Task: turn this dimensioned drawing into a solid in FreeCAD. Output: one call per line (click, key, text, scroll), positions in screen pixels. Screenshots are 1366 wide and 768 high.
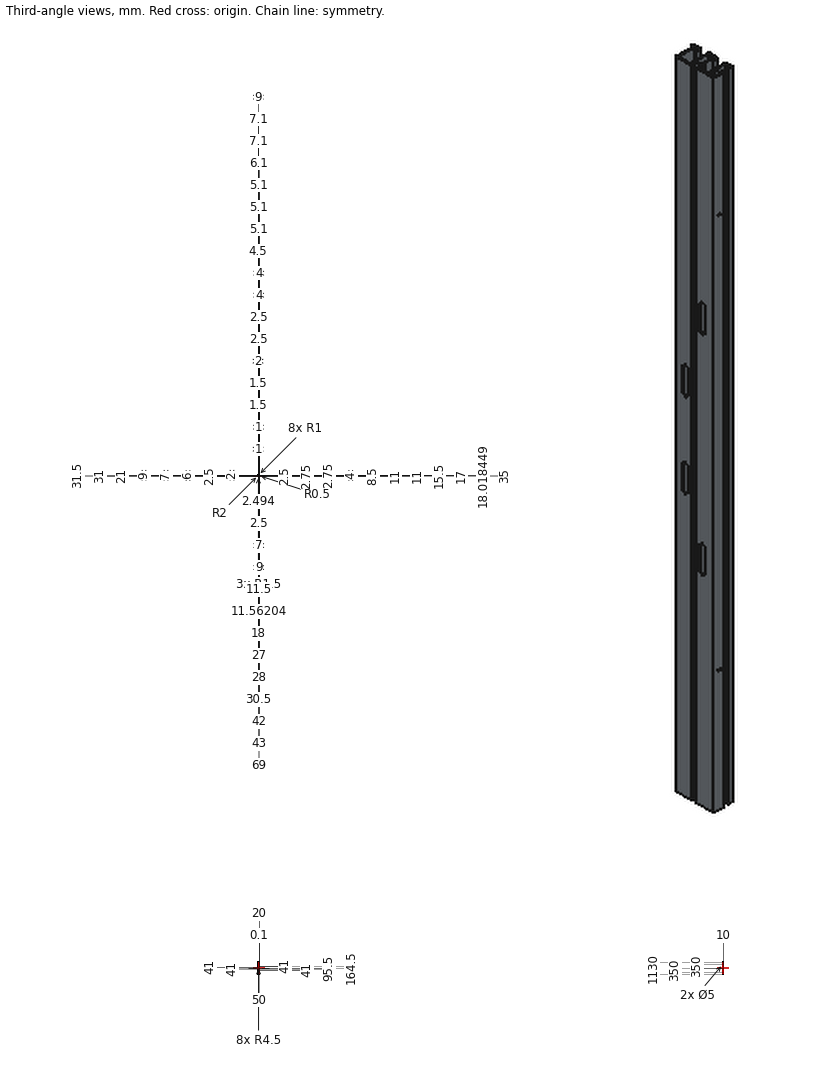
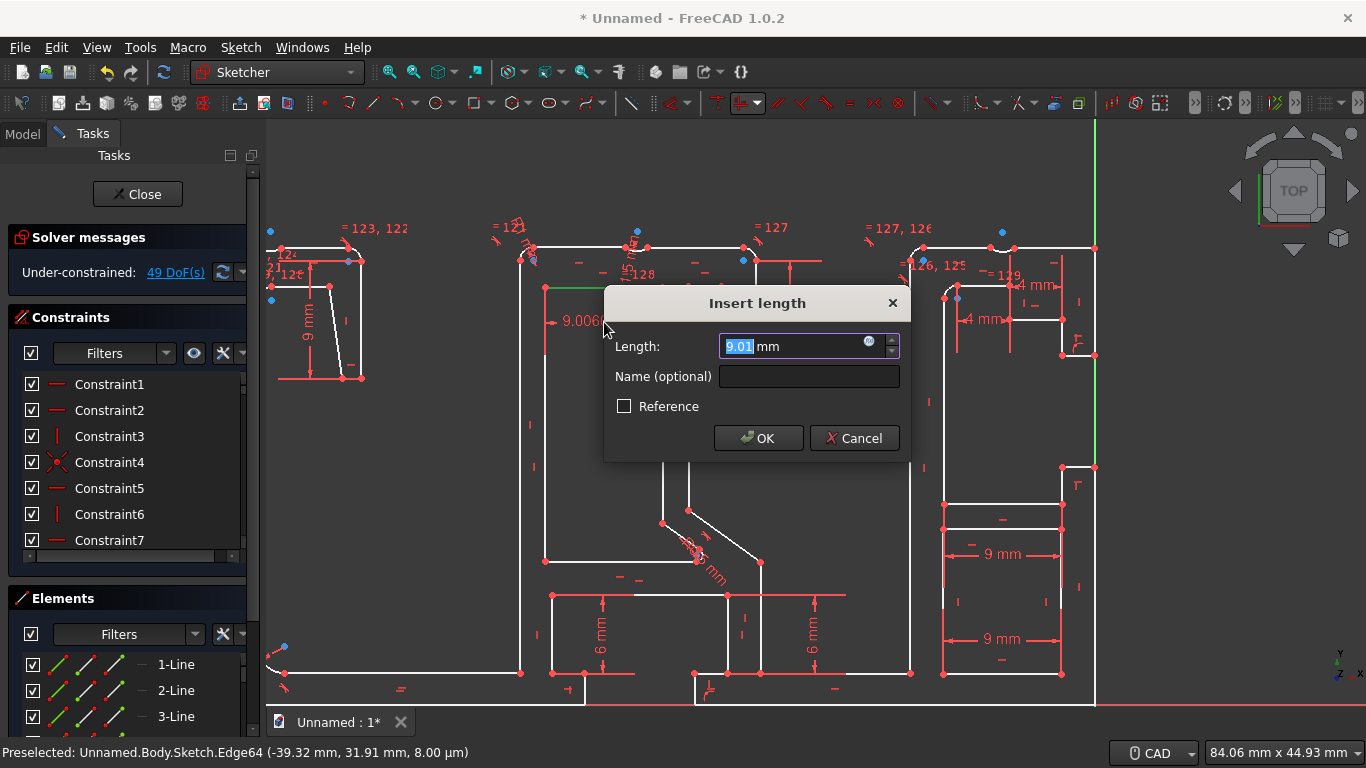
text(9)
key(Return)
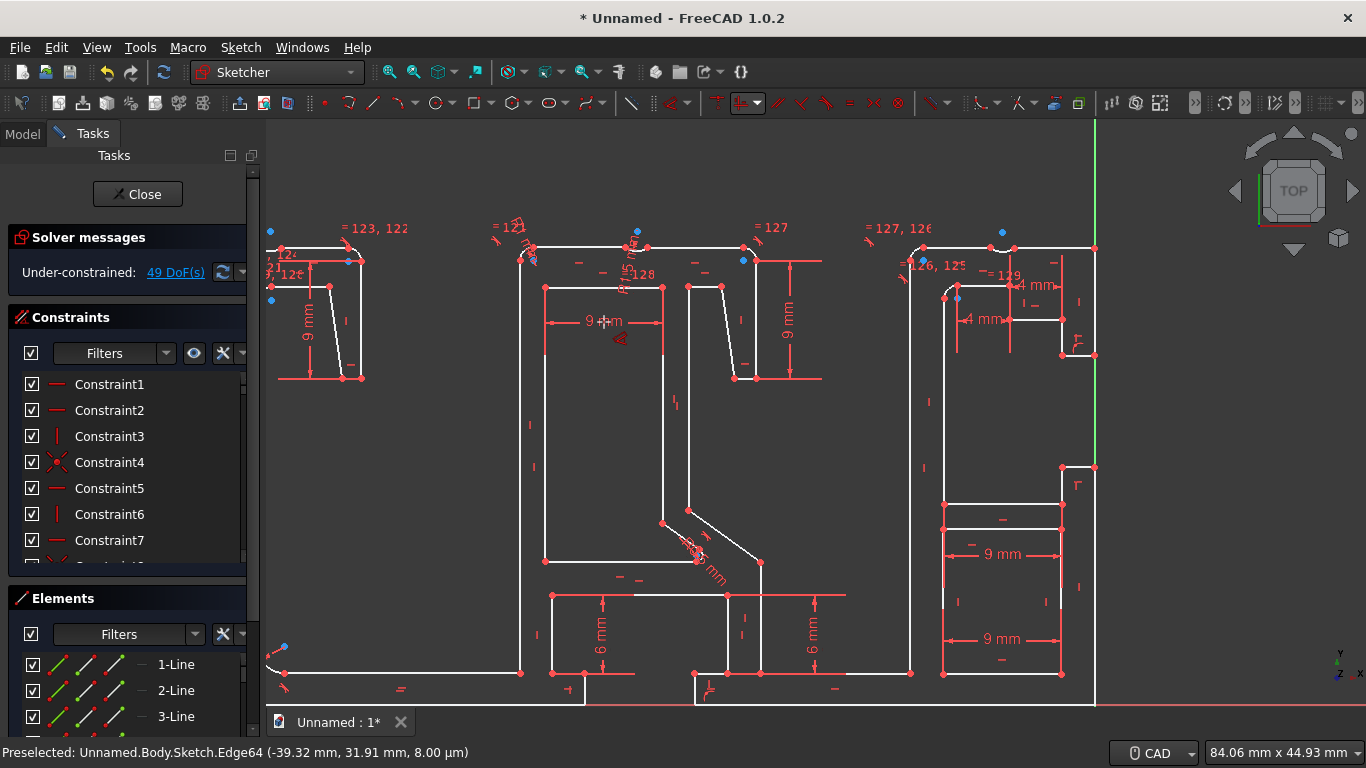
click(449, 673)
click(407, 639)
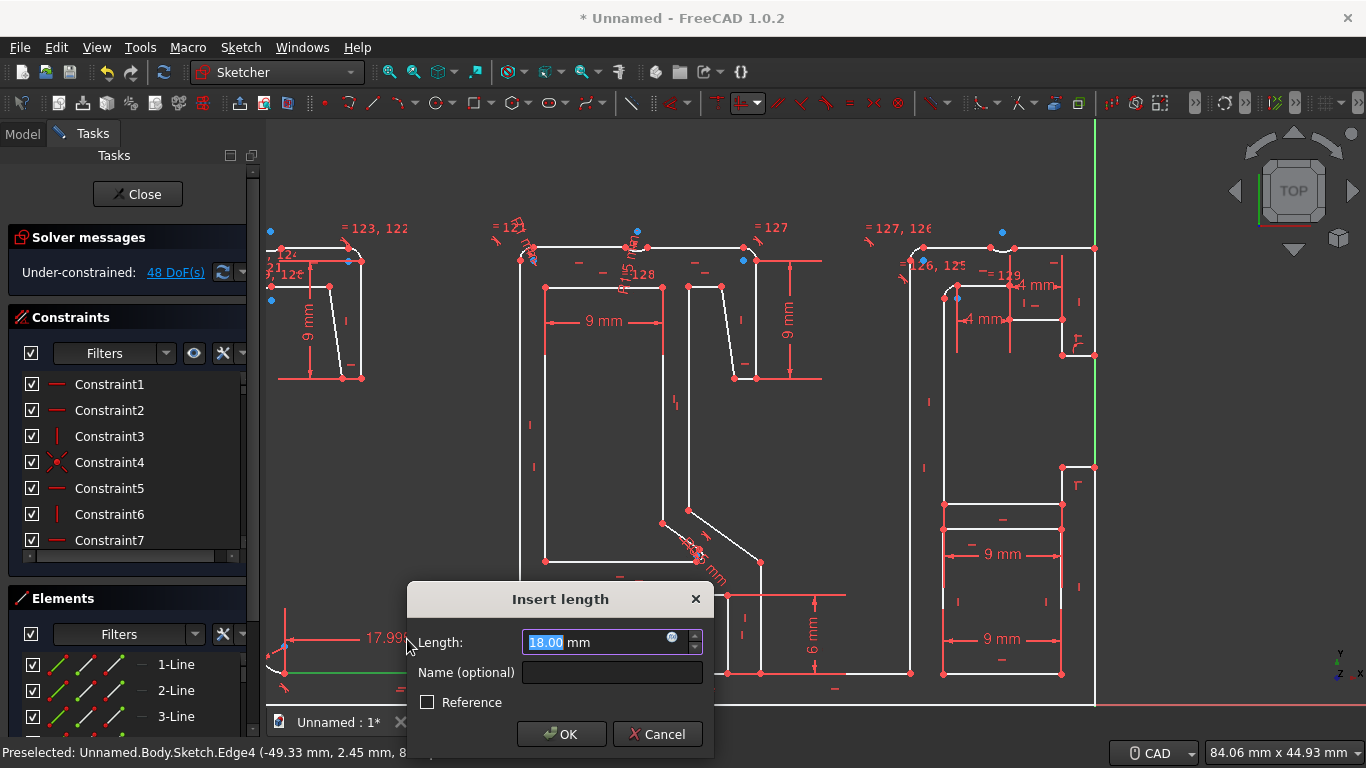
text(18)
key(Return)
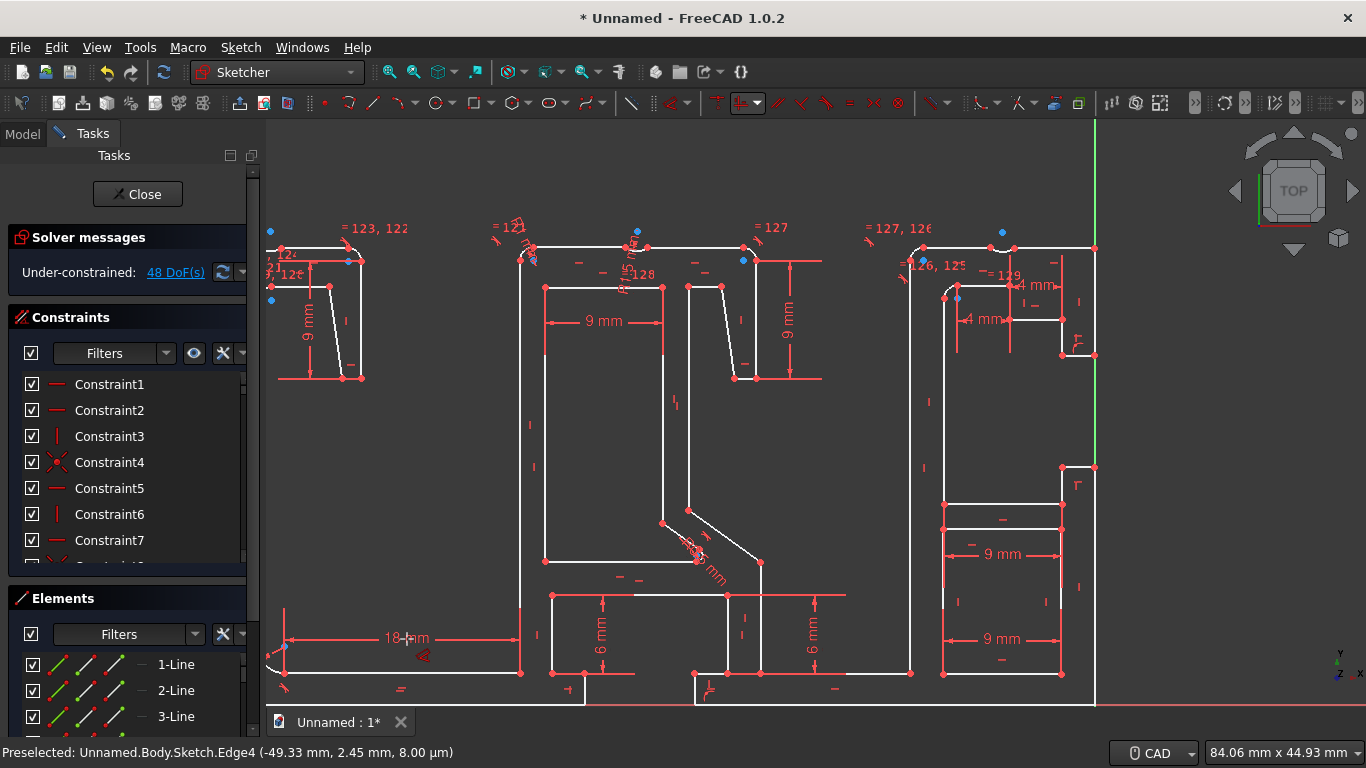
scroll(973, 284, down, 2)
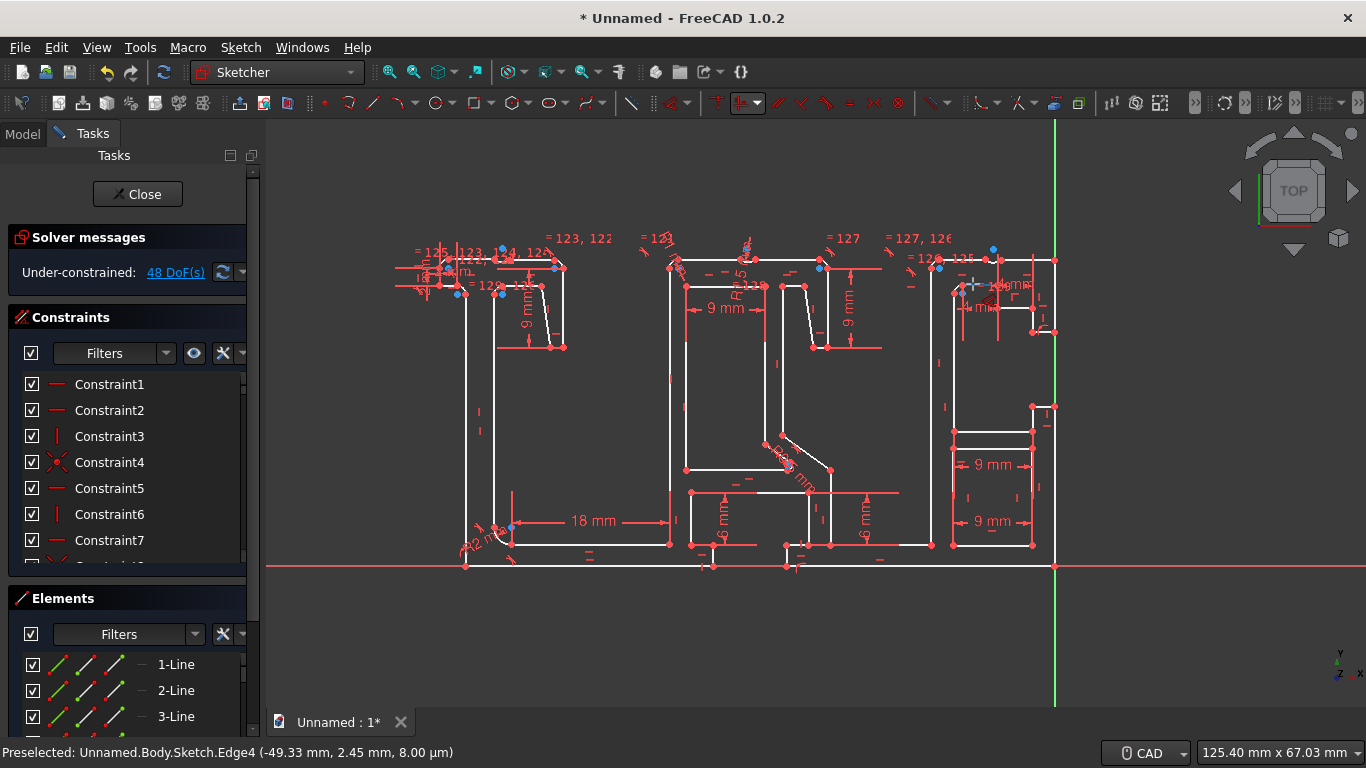
click(466, 376)
click(432, 430)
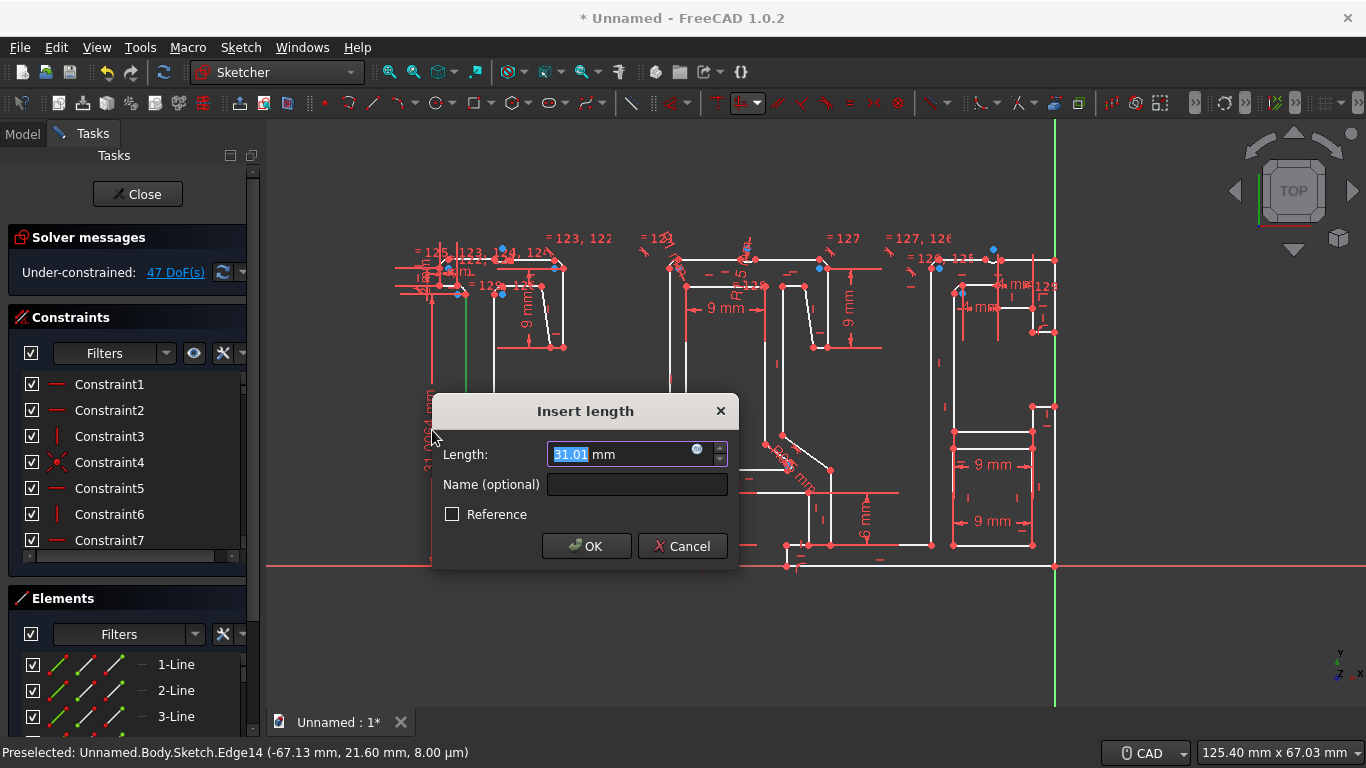
text(31)
key(Return)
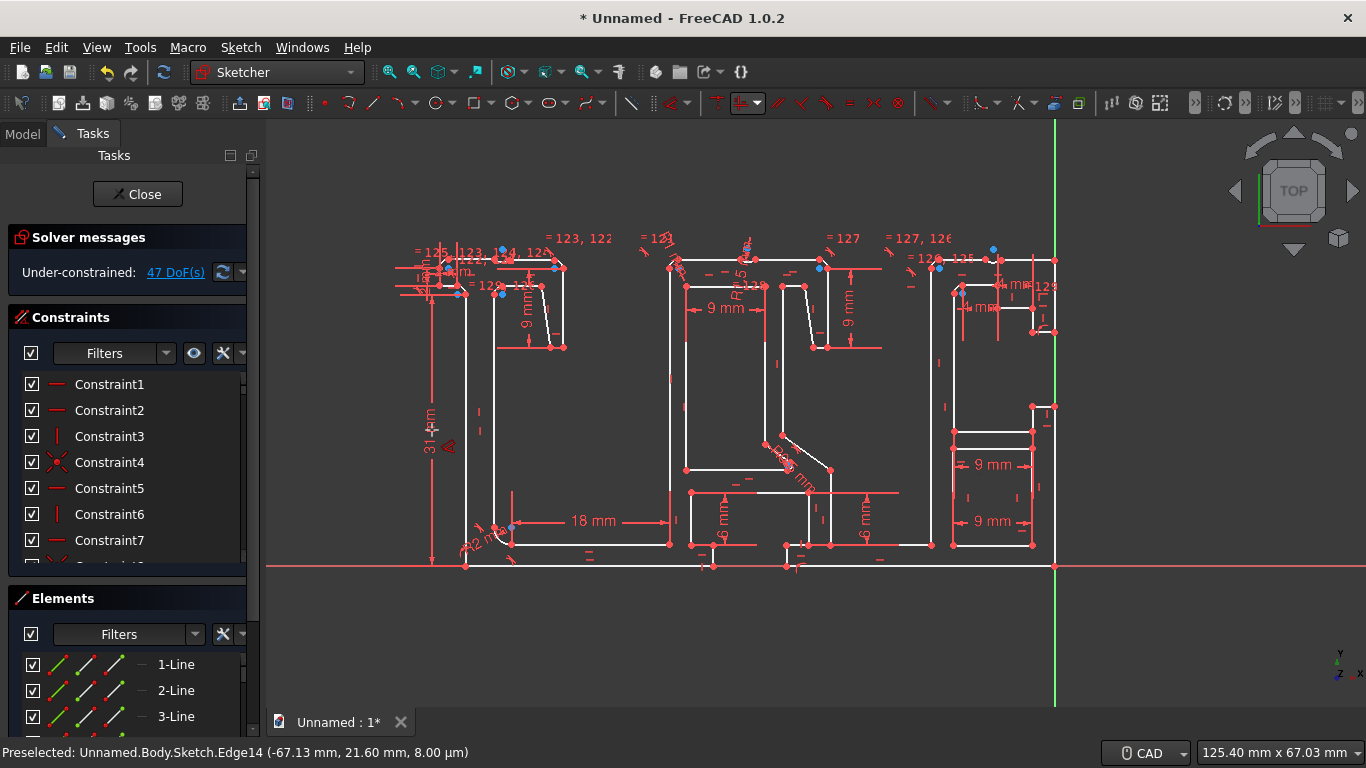
click(540, 566)
click(589, 600)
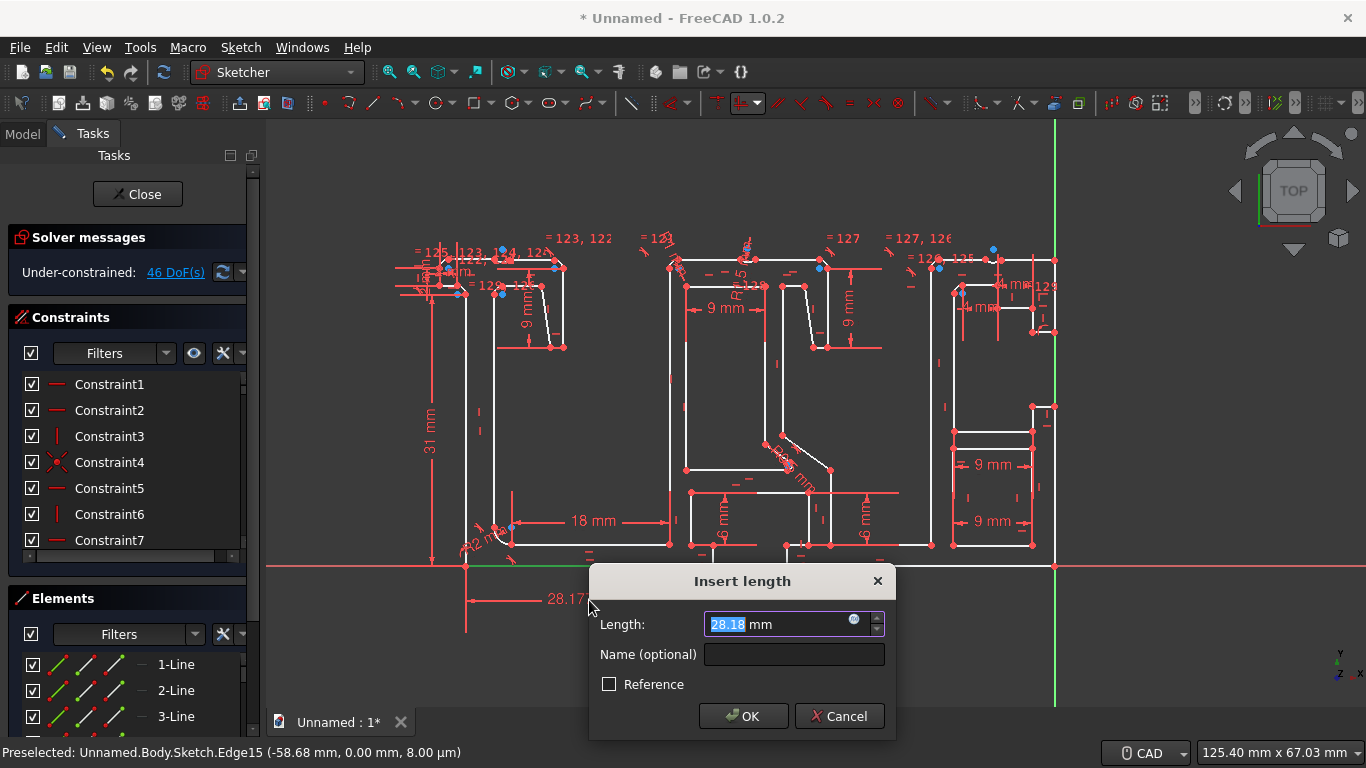
text(28)
key(Return)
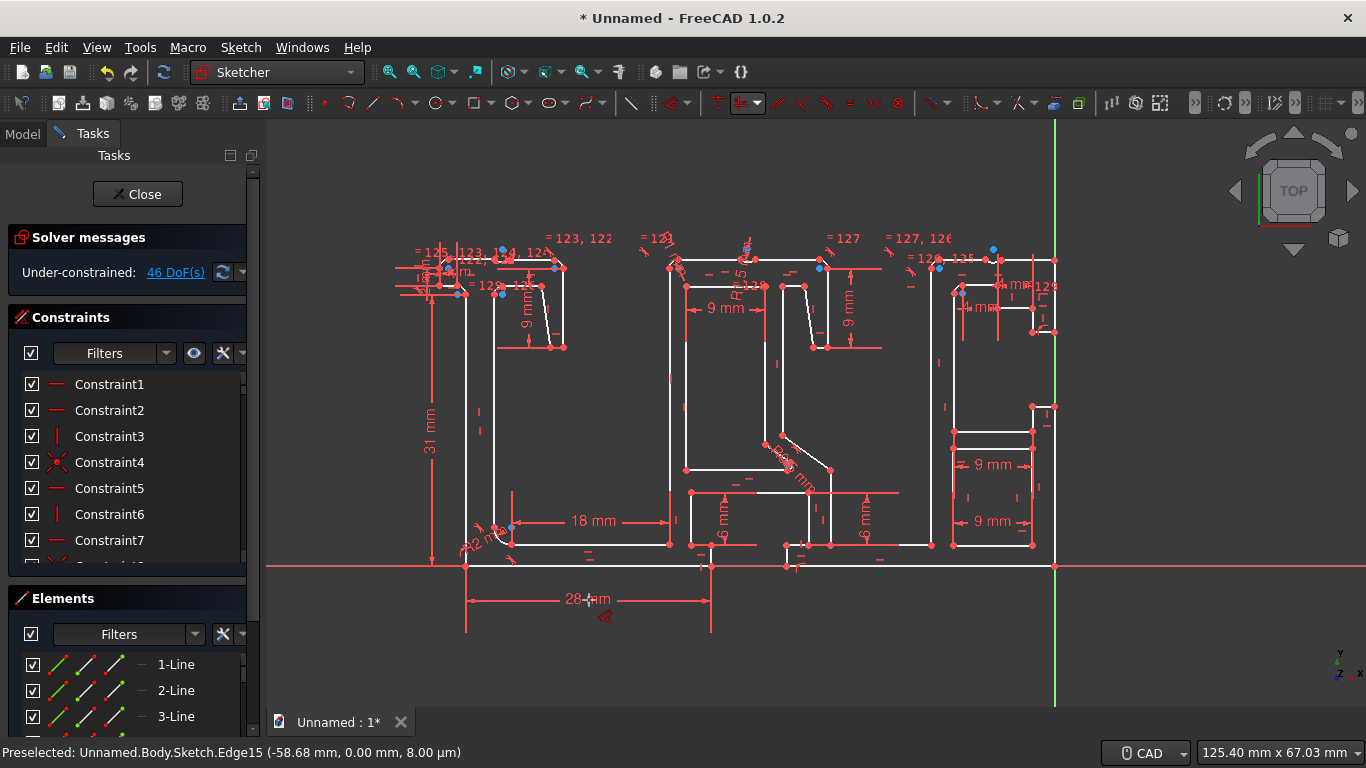
click(783, 391)
click(817, 361)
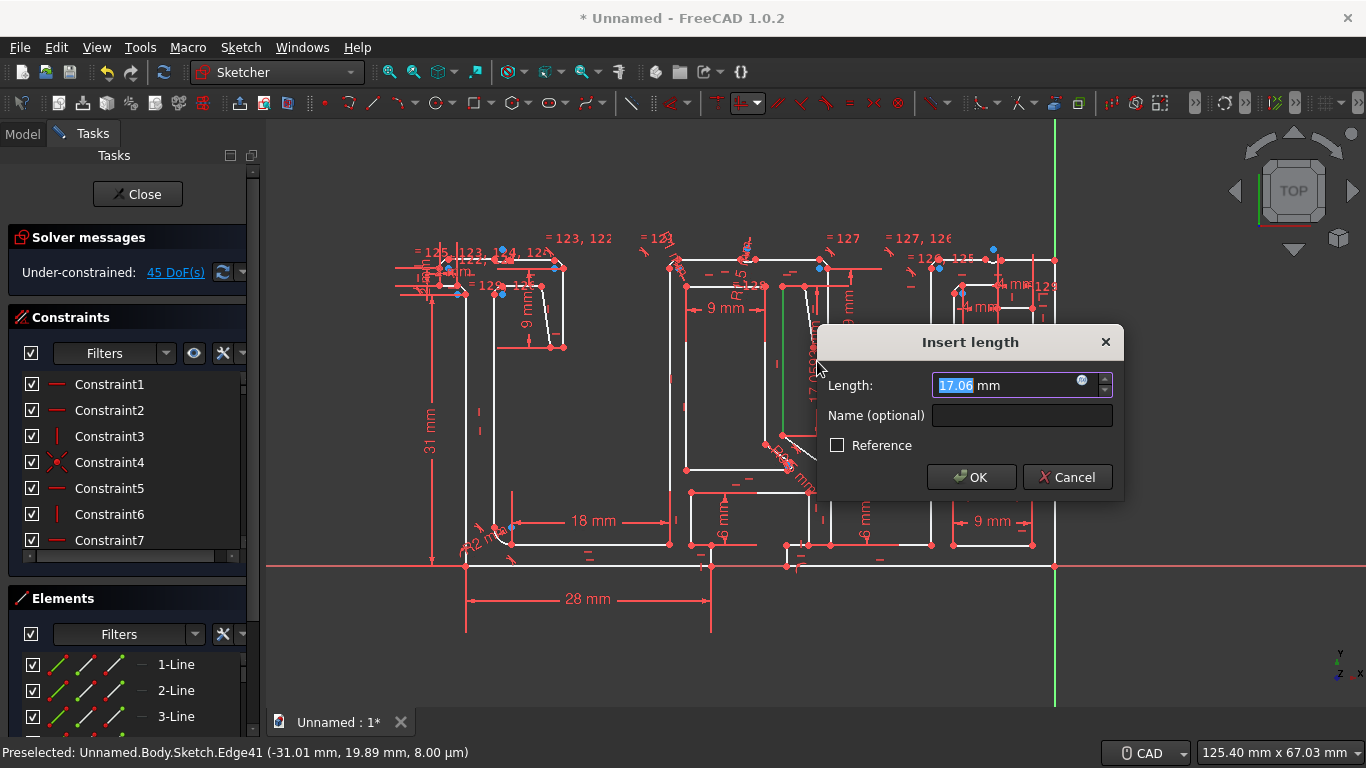
text(17)
key(Return)